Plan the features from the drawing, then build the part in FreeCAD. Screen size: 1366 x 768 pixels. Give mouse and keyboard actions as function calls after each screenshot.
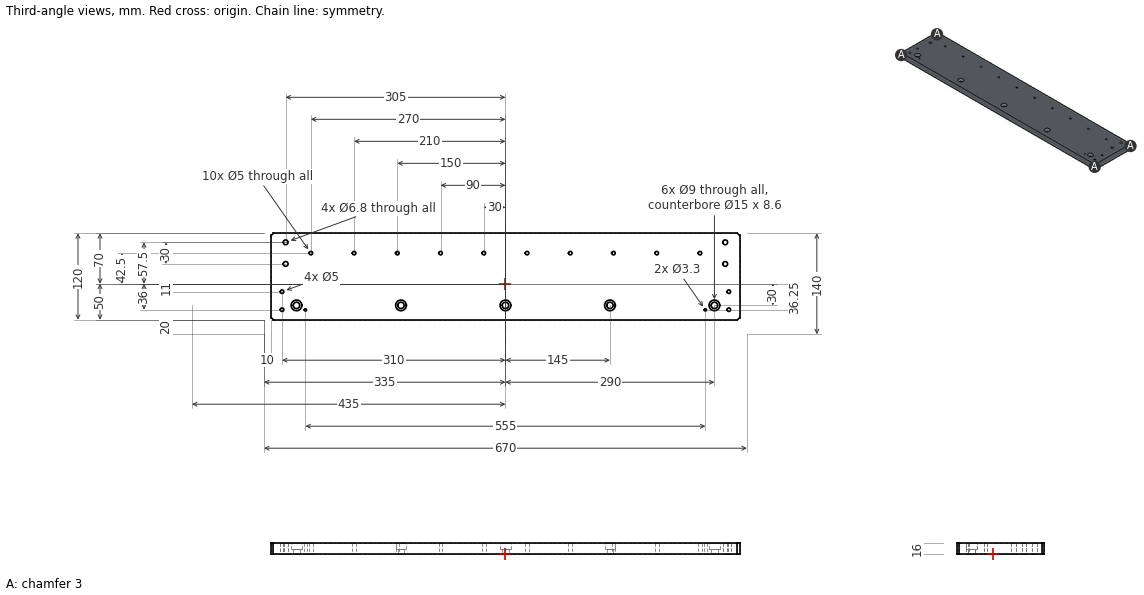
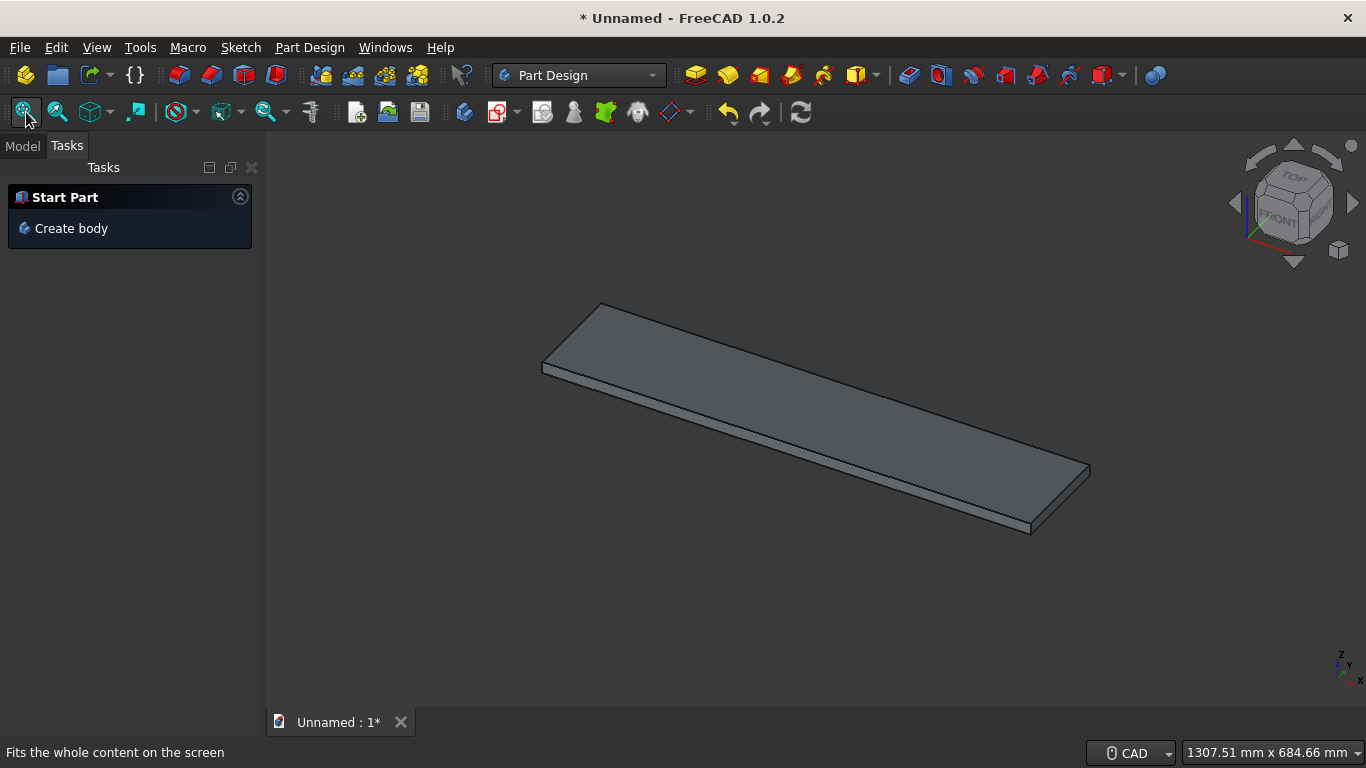
click(955, 459)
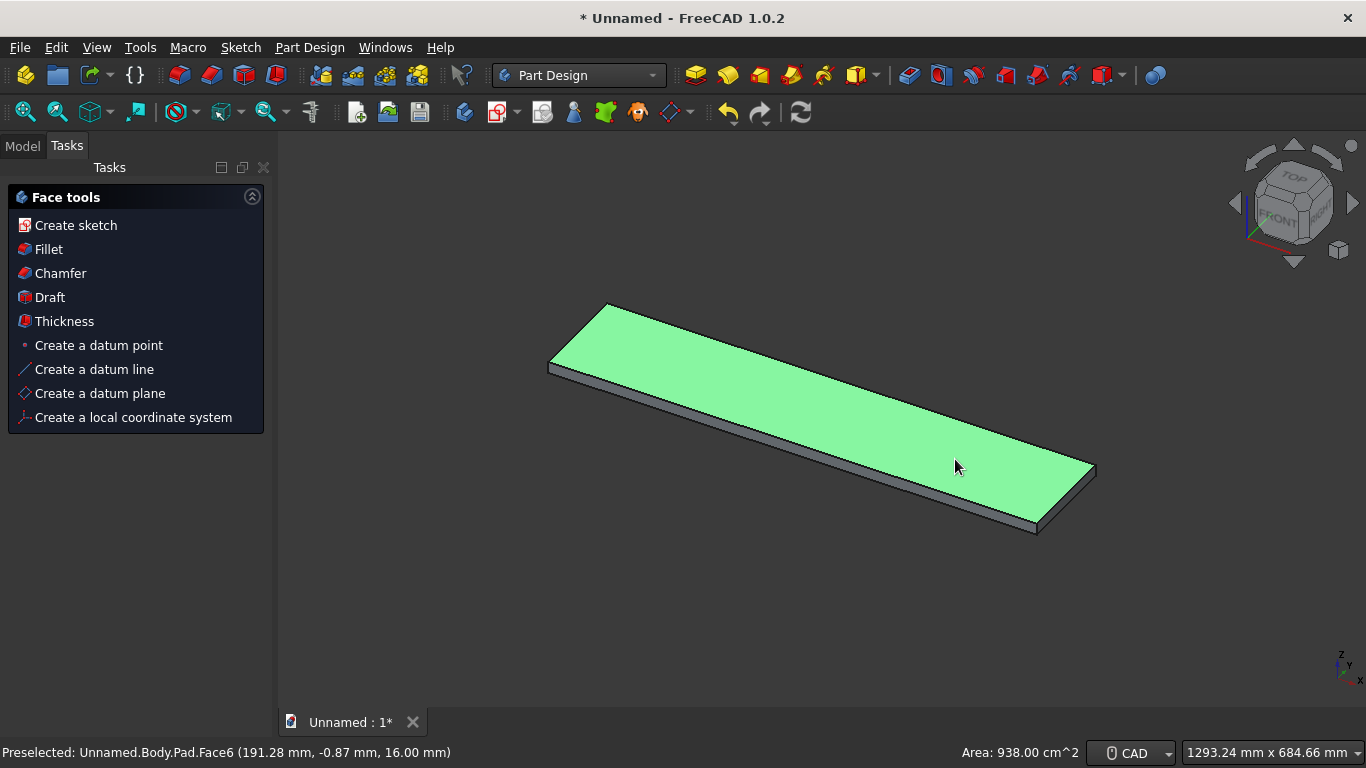
click(498, 112)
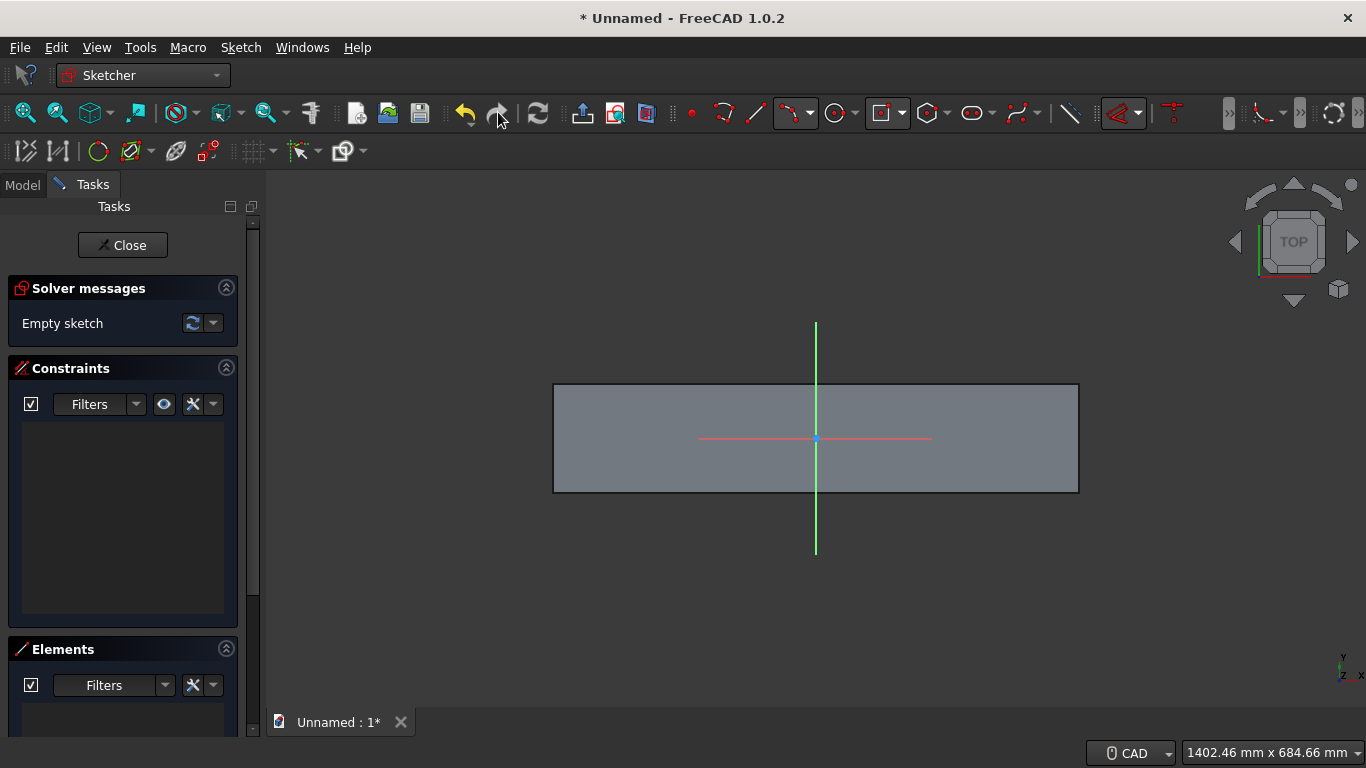
click(836, 114)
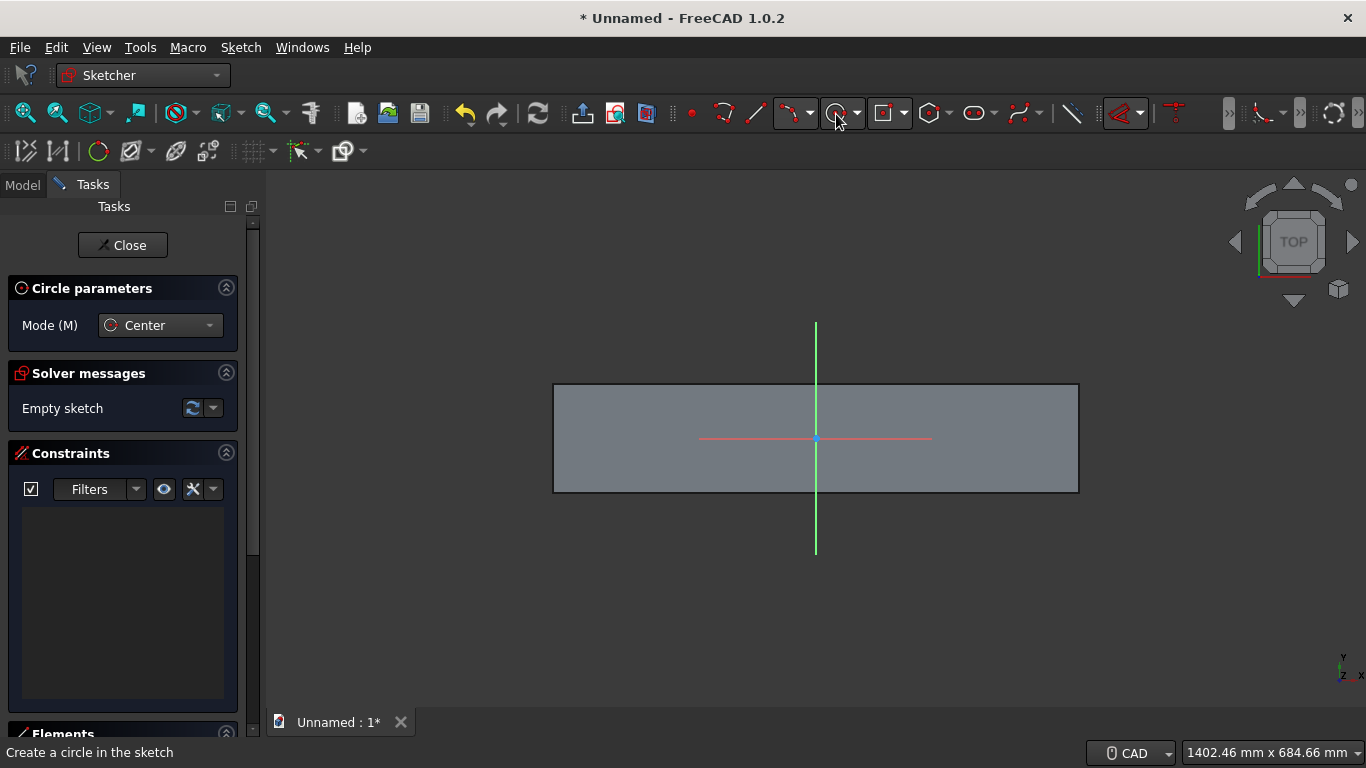
scroll(577, 393, up, 11)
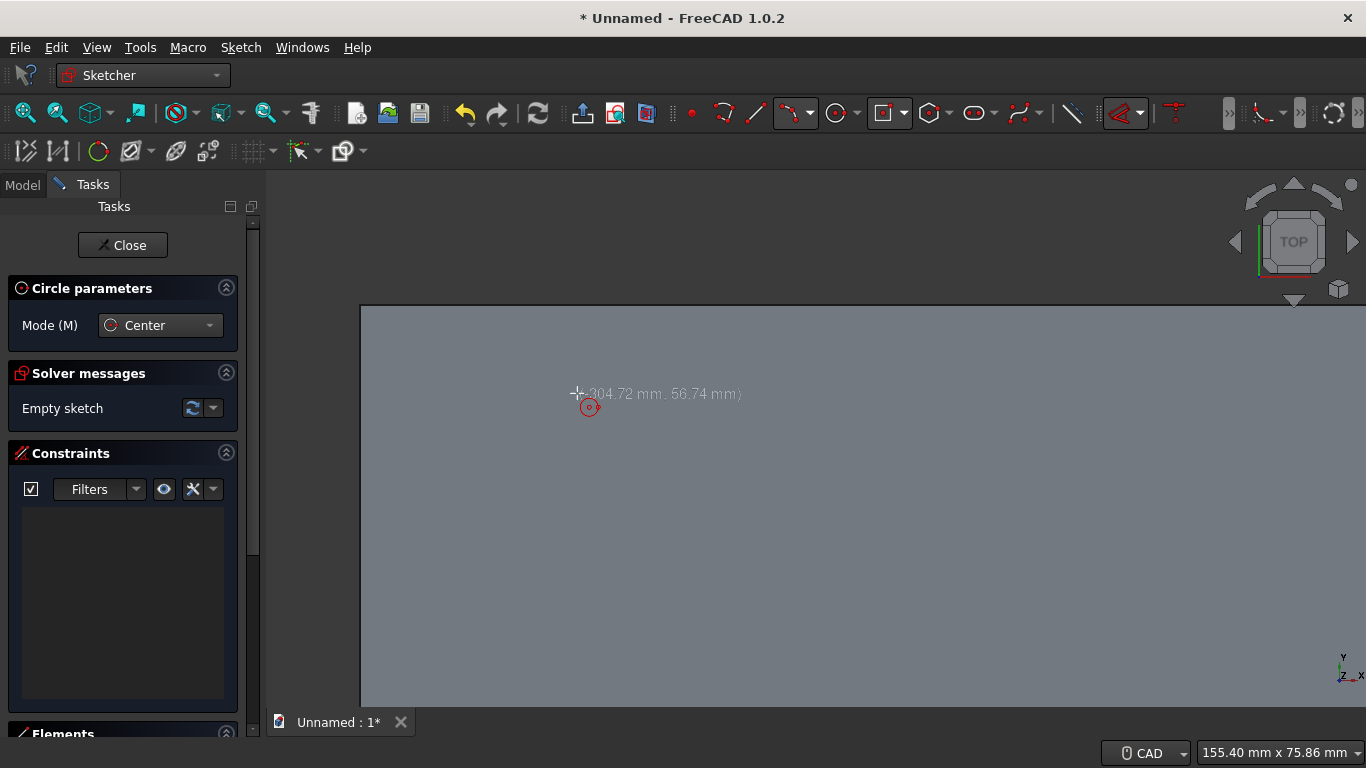
scroll(437, 416, down, 10)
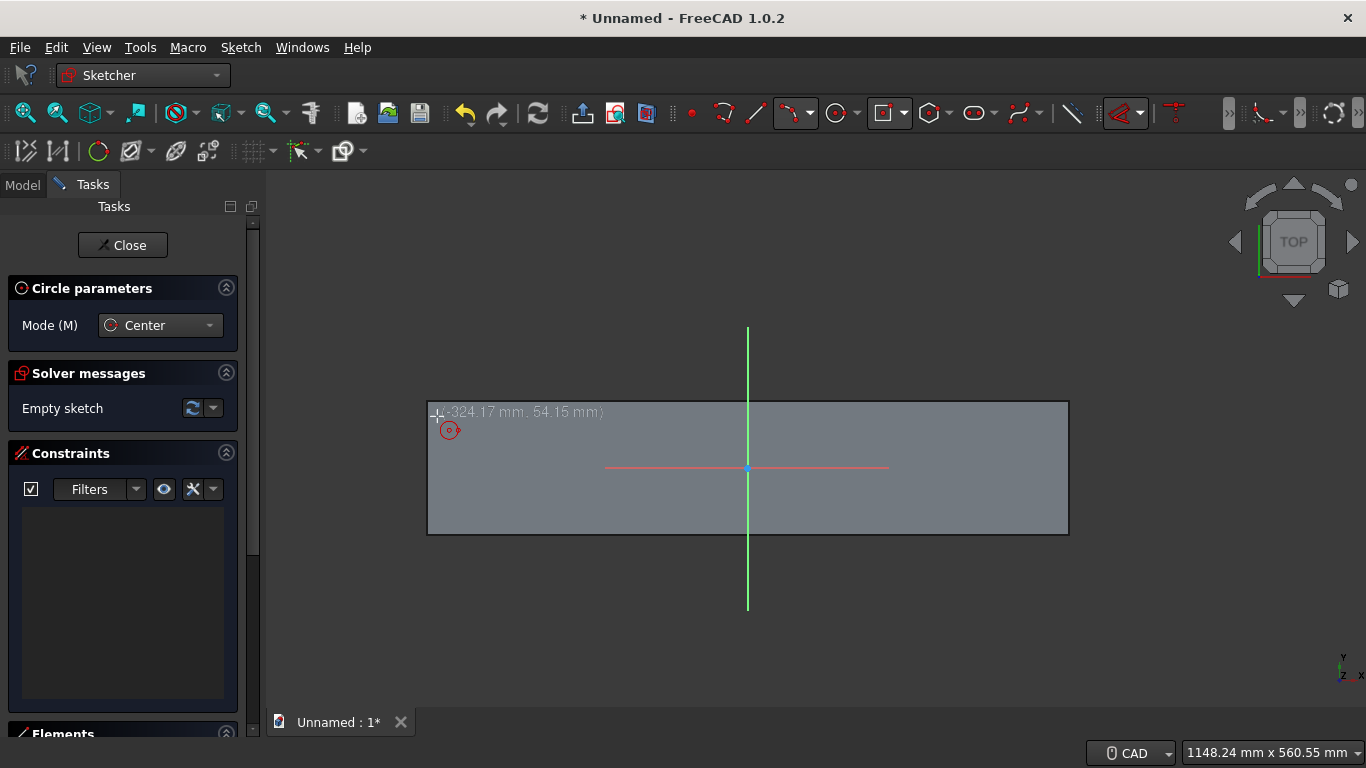
click(456, 413)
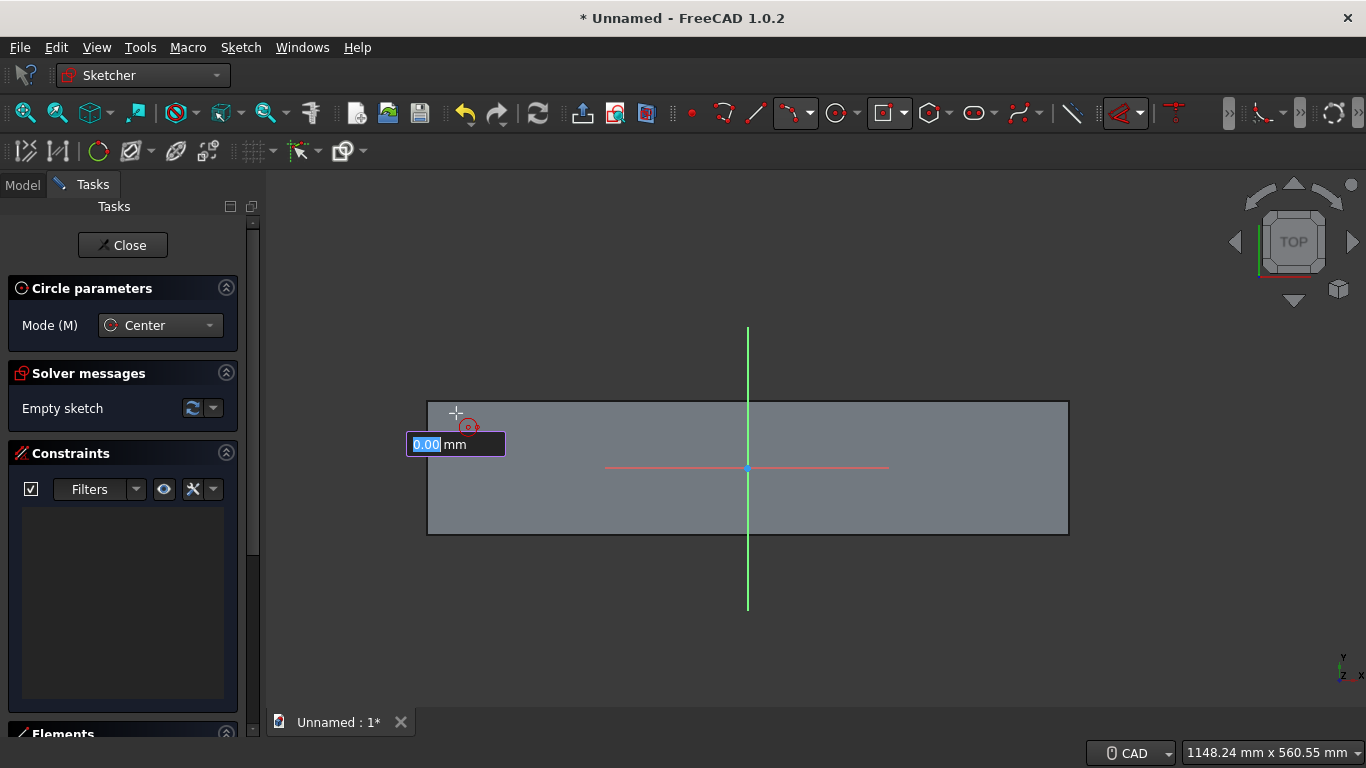
scroll(458, 411, up, 8)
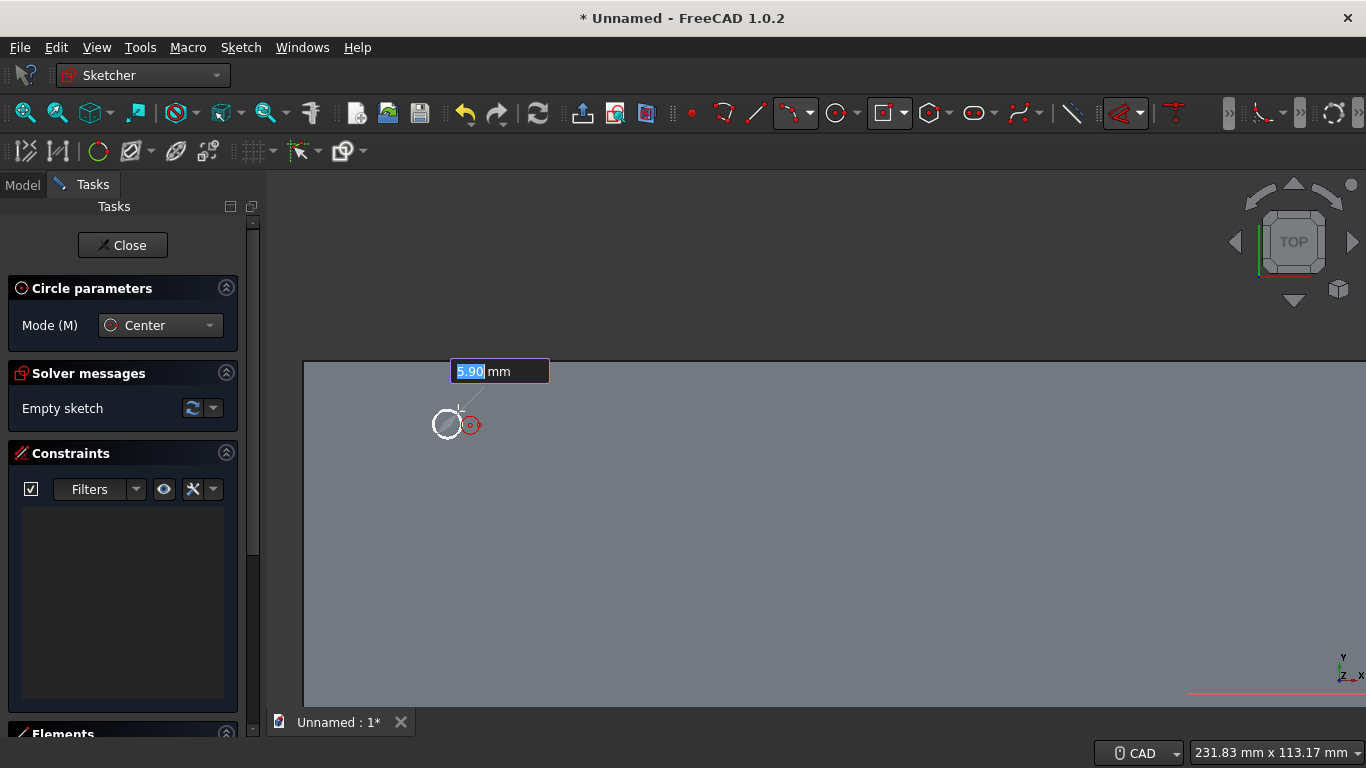
click(456, 409)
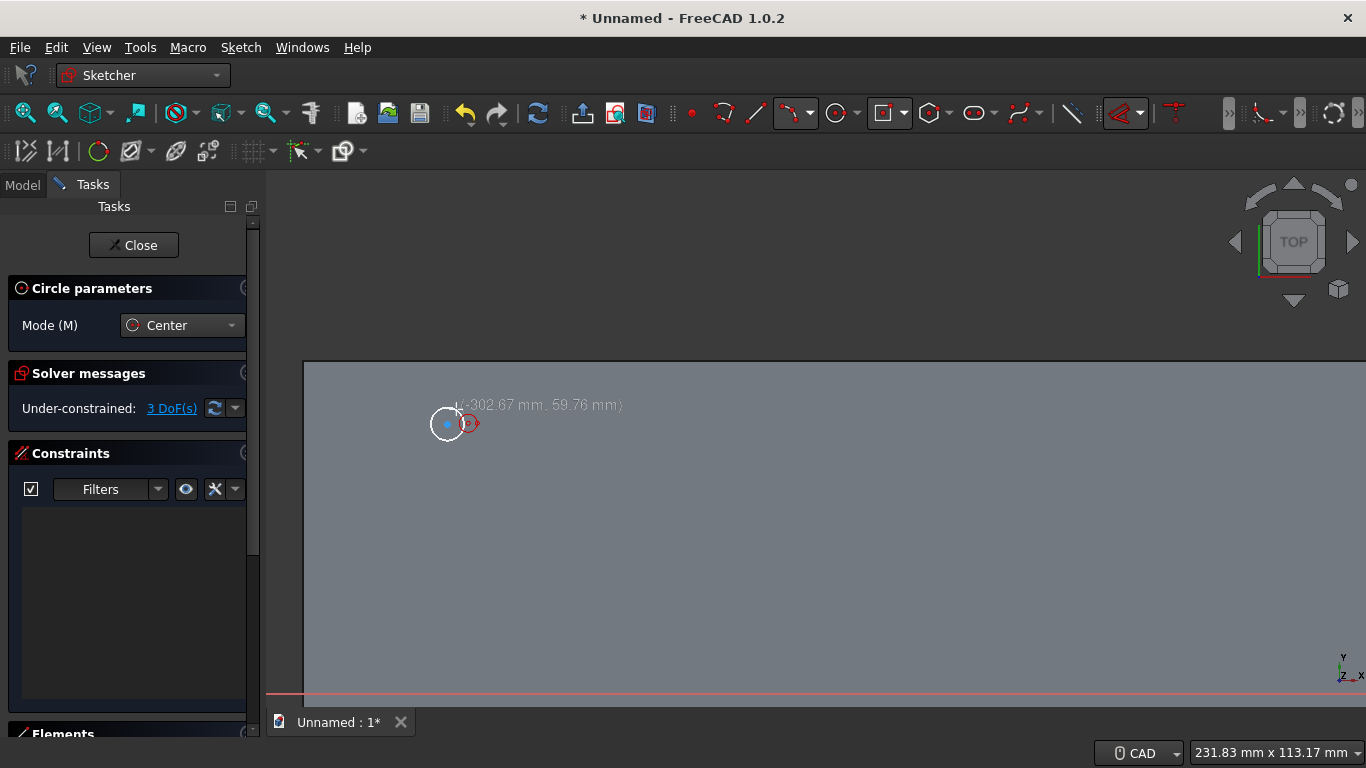
scroll(445, 563, up, 2)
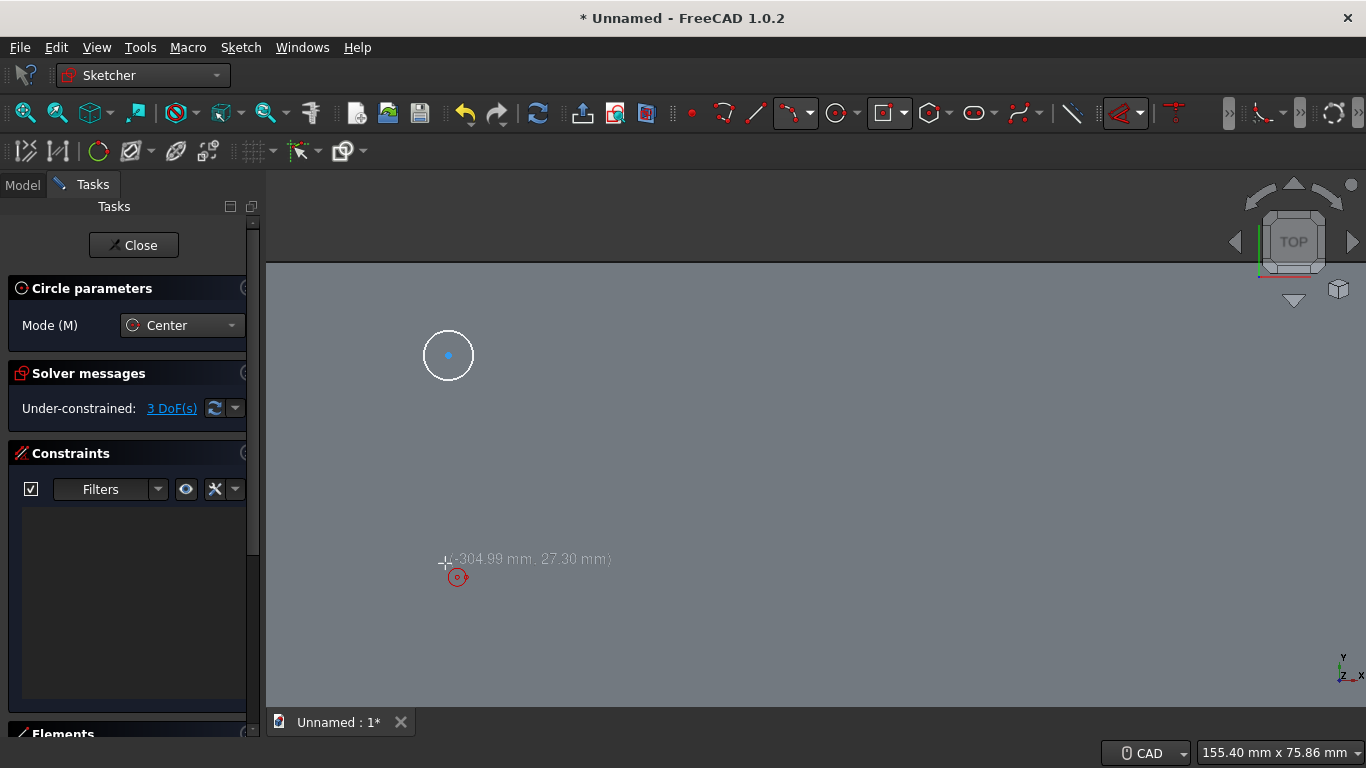
scroll(457, 422, down, 10)